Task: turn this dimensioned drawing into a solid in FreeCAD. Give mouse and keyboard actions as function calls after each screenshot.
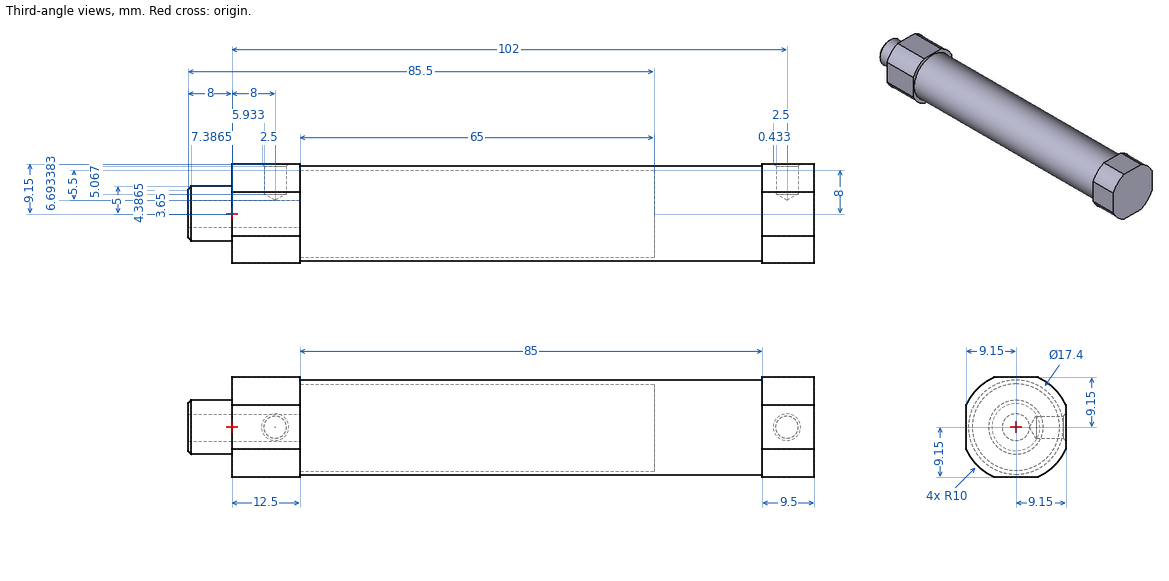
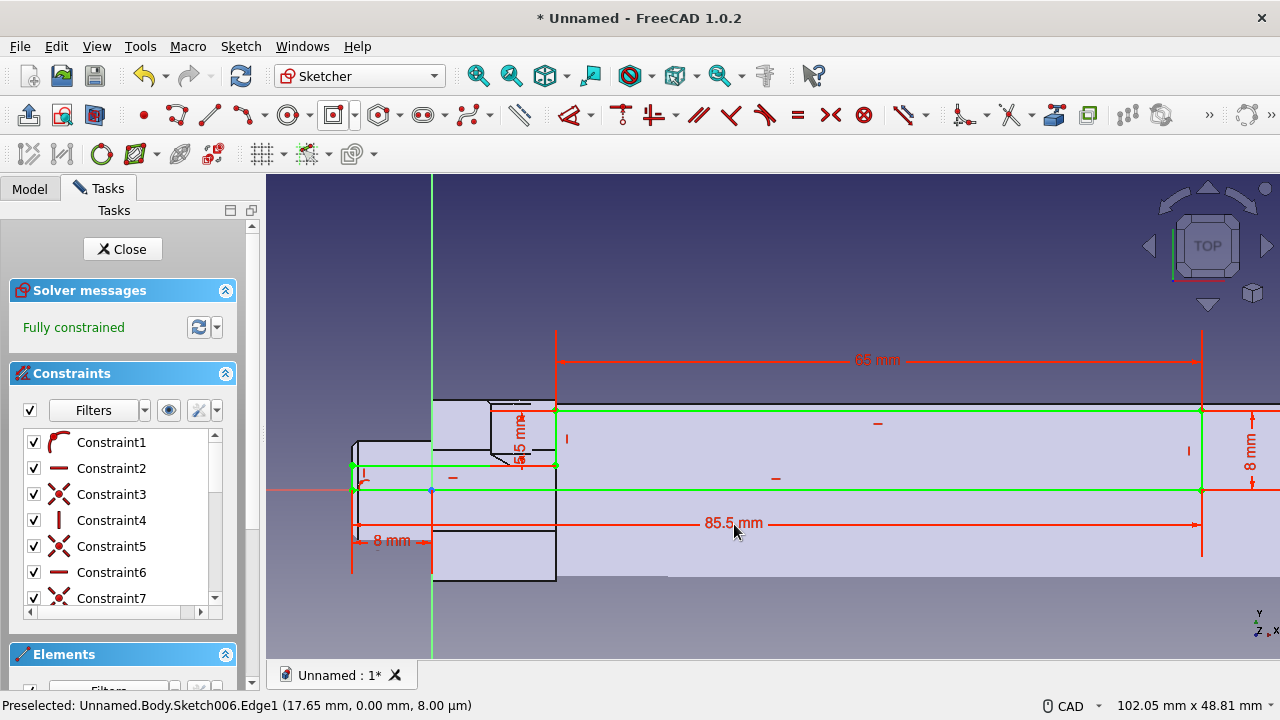
click(123, 249)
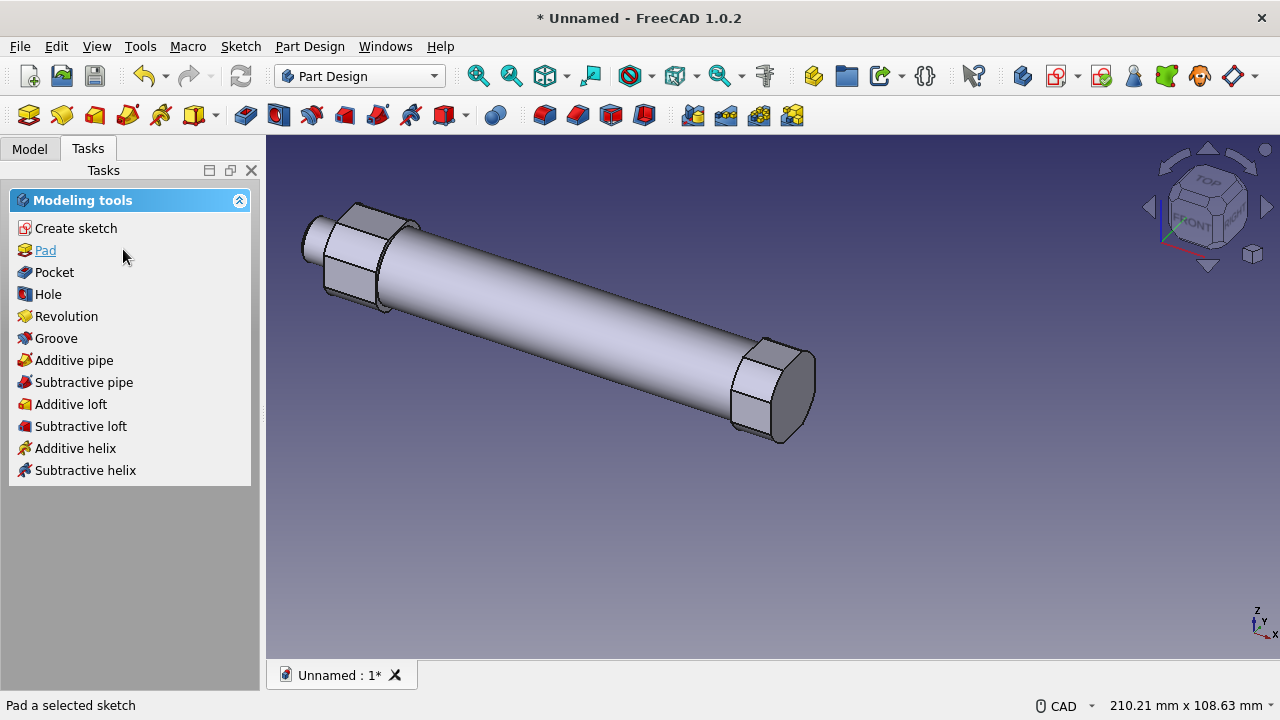
click(312, 116)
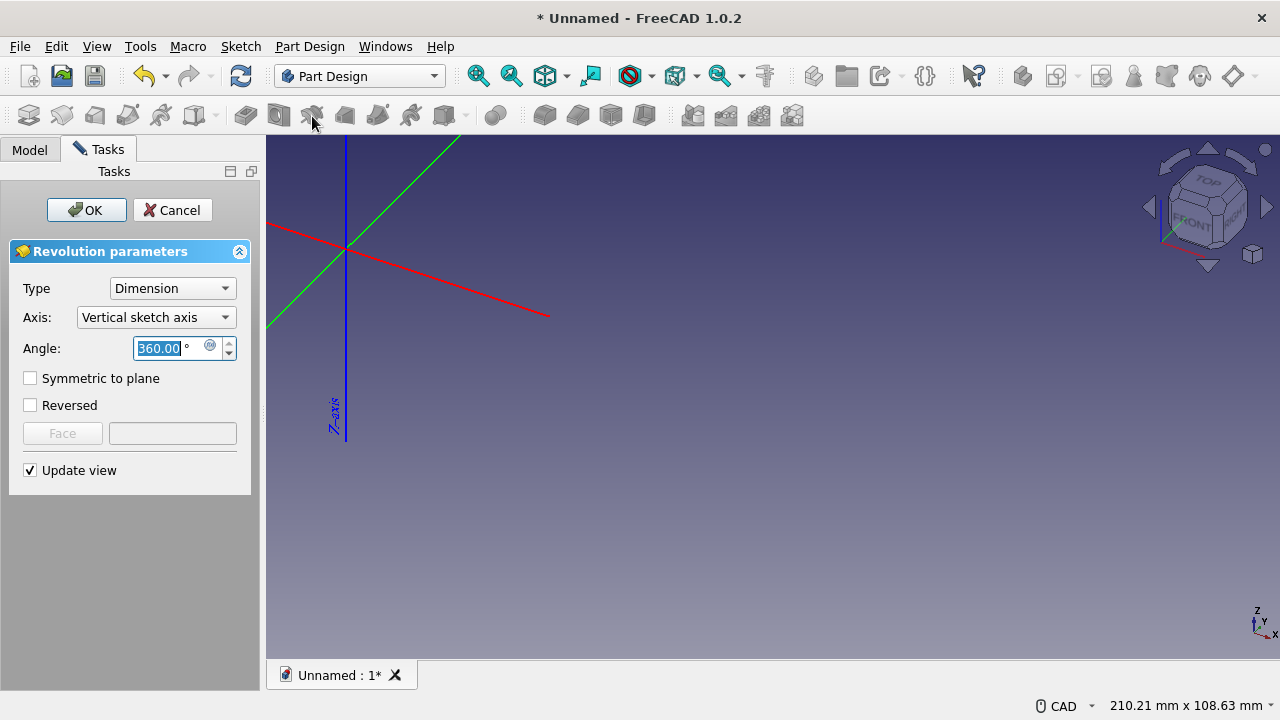
click(157, 318)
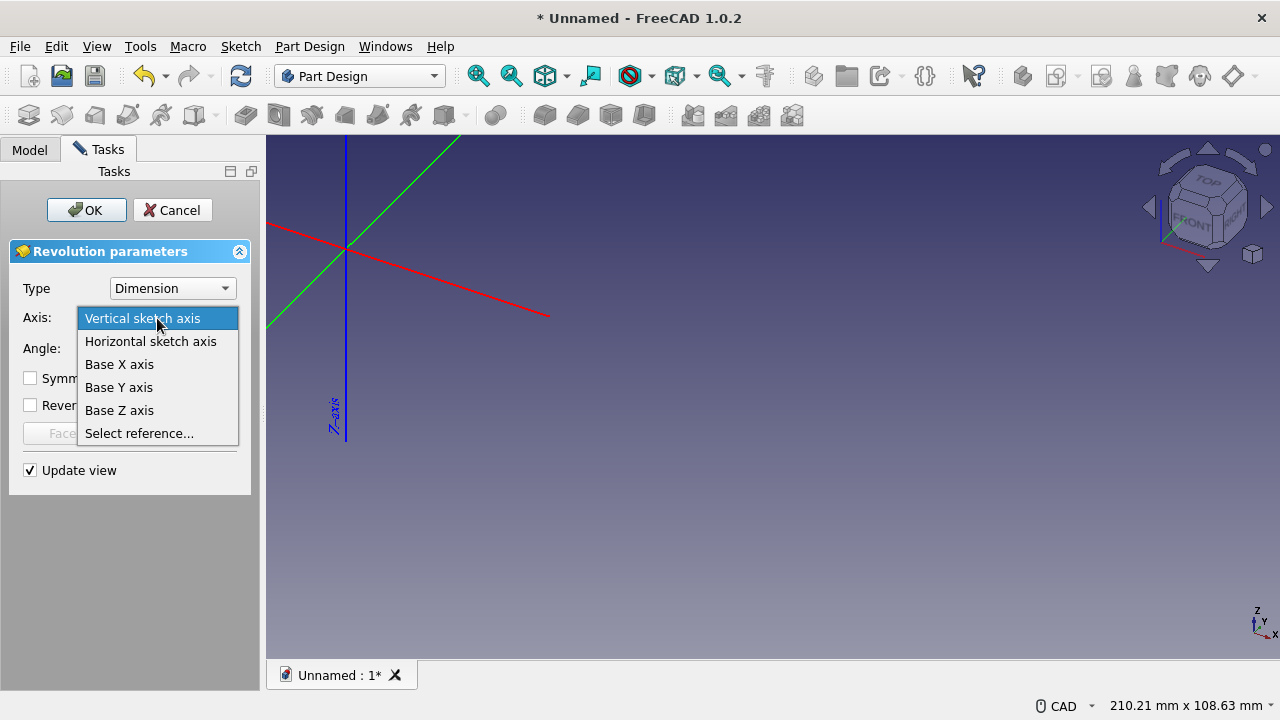
click(156, 342)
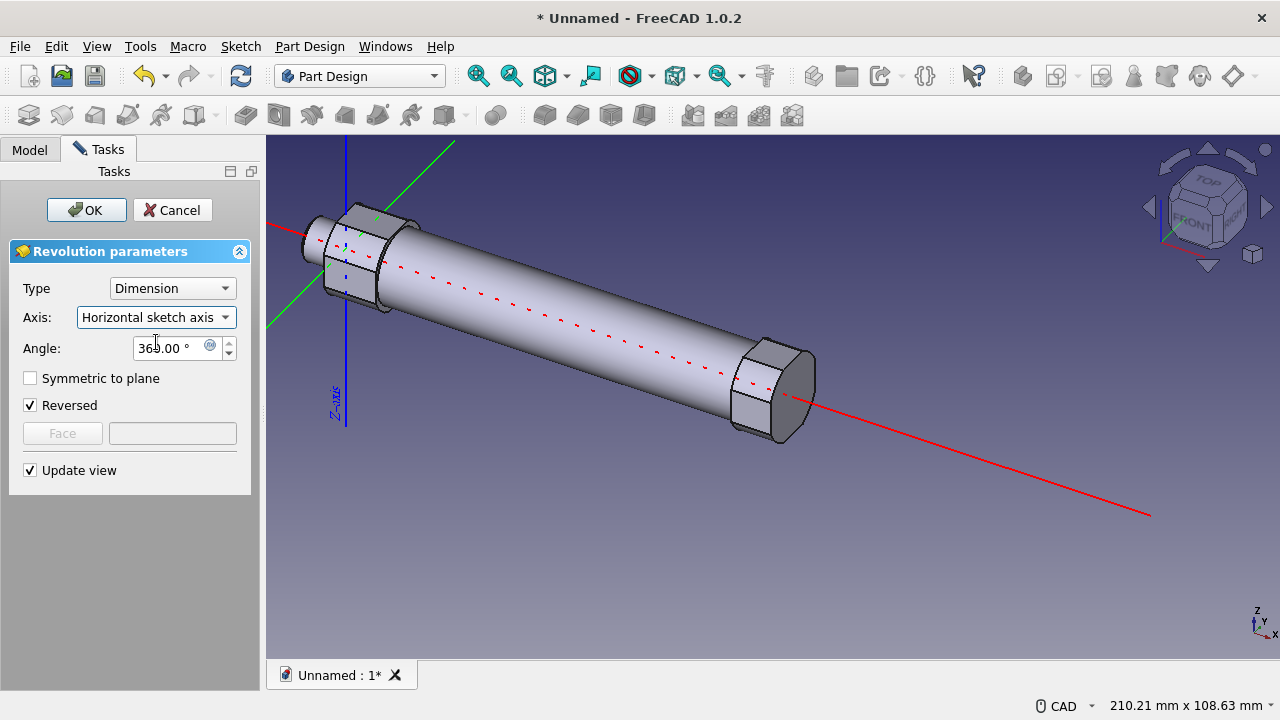
click(87, 210)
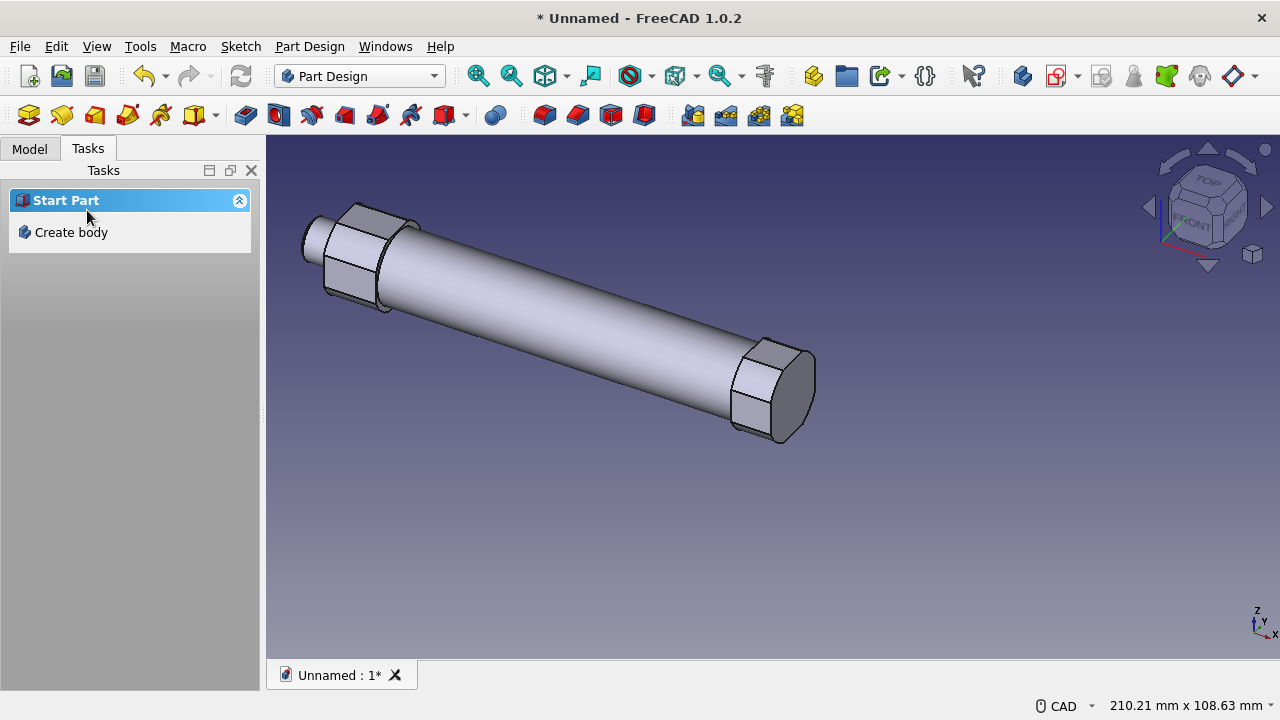
key(0)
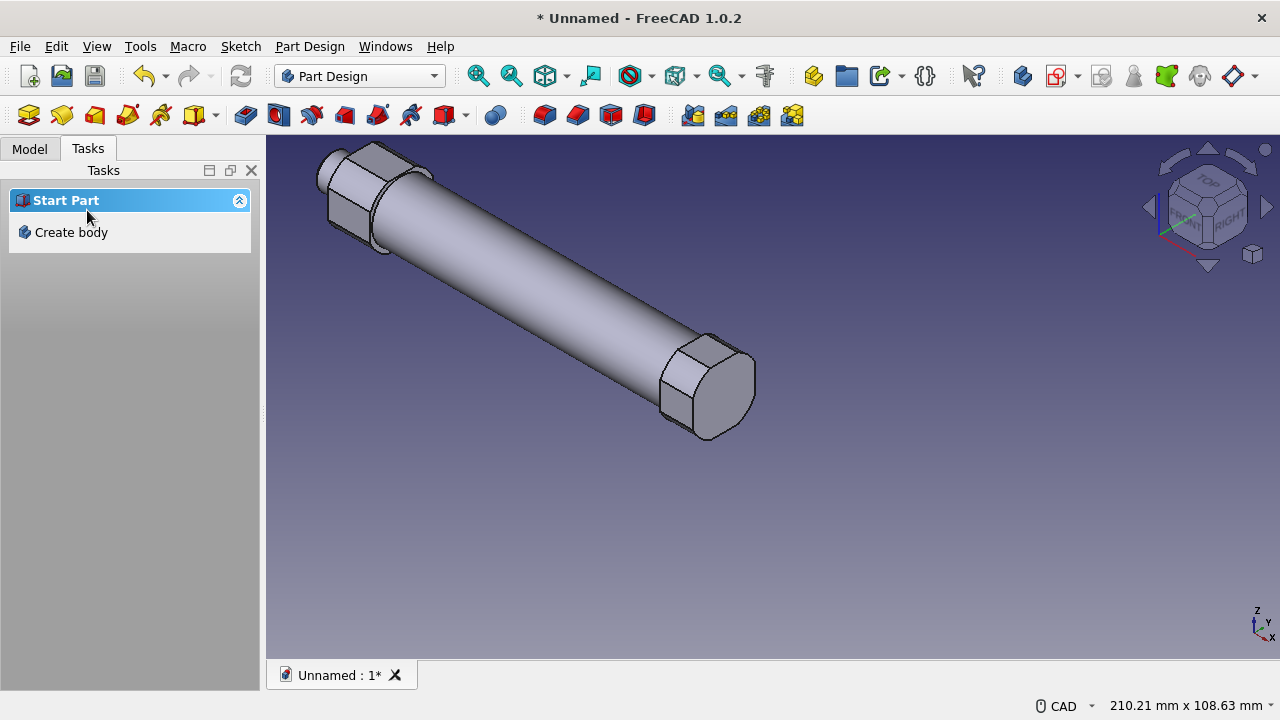
click(479, 76)